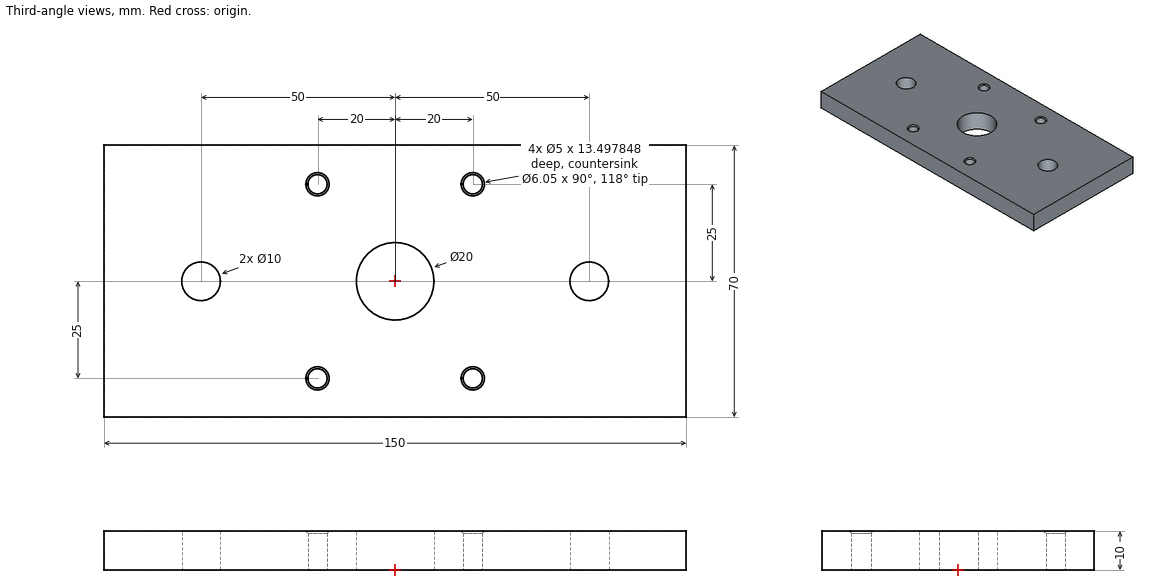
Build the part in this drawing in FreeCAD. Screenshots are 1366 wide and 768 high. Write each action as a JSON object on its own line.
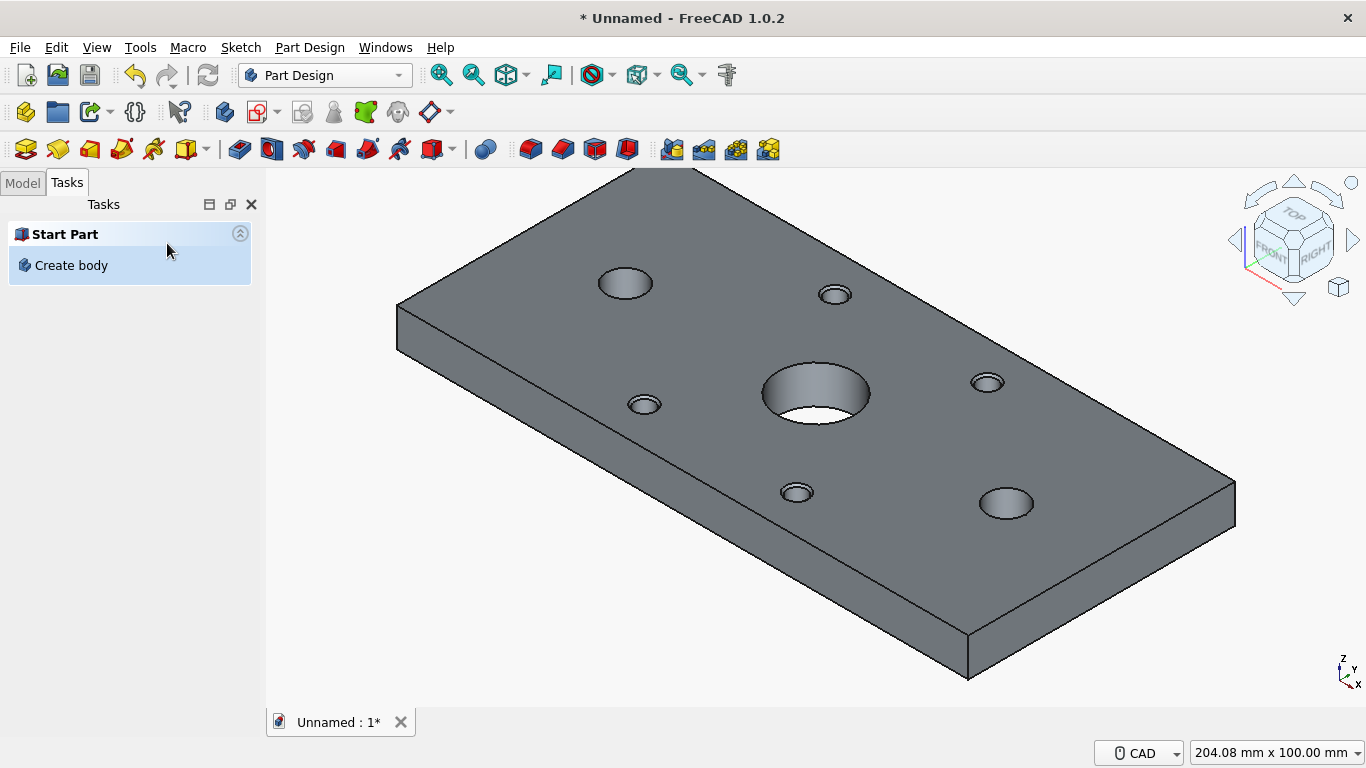
{"action": "left_click", "coordinate": [442, 76]}